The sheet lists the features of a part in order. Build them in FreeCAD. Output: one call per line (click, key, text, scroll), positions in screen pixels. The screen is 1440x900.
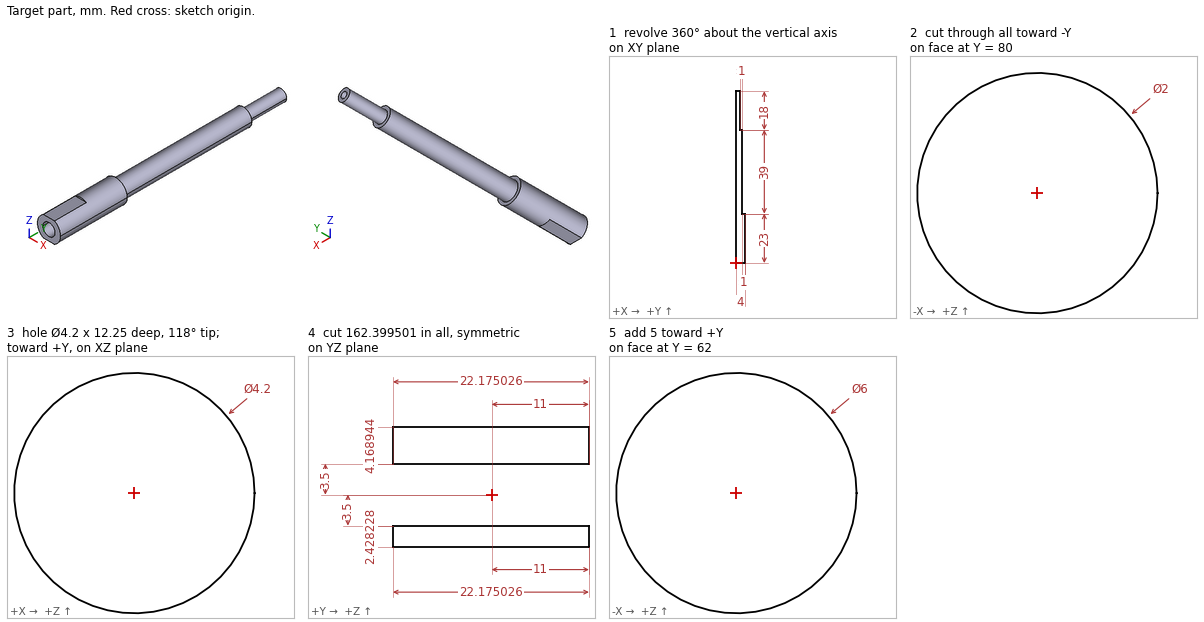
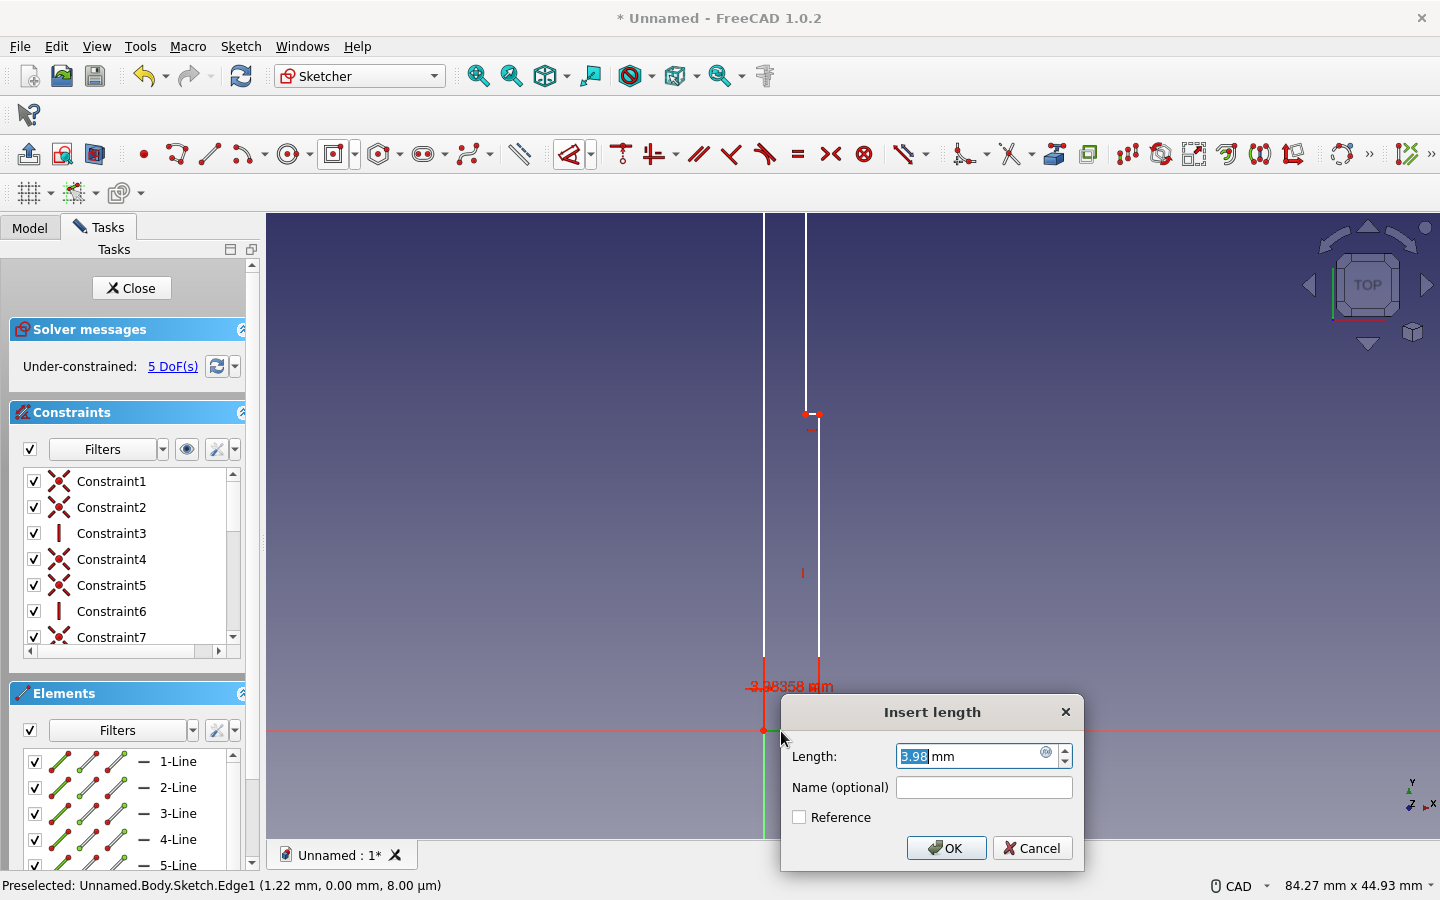
text(4)
key(Return)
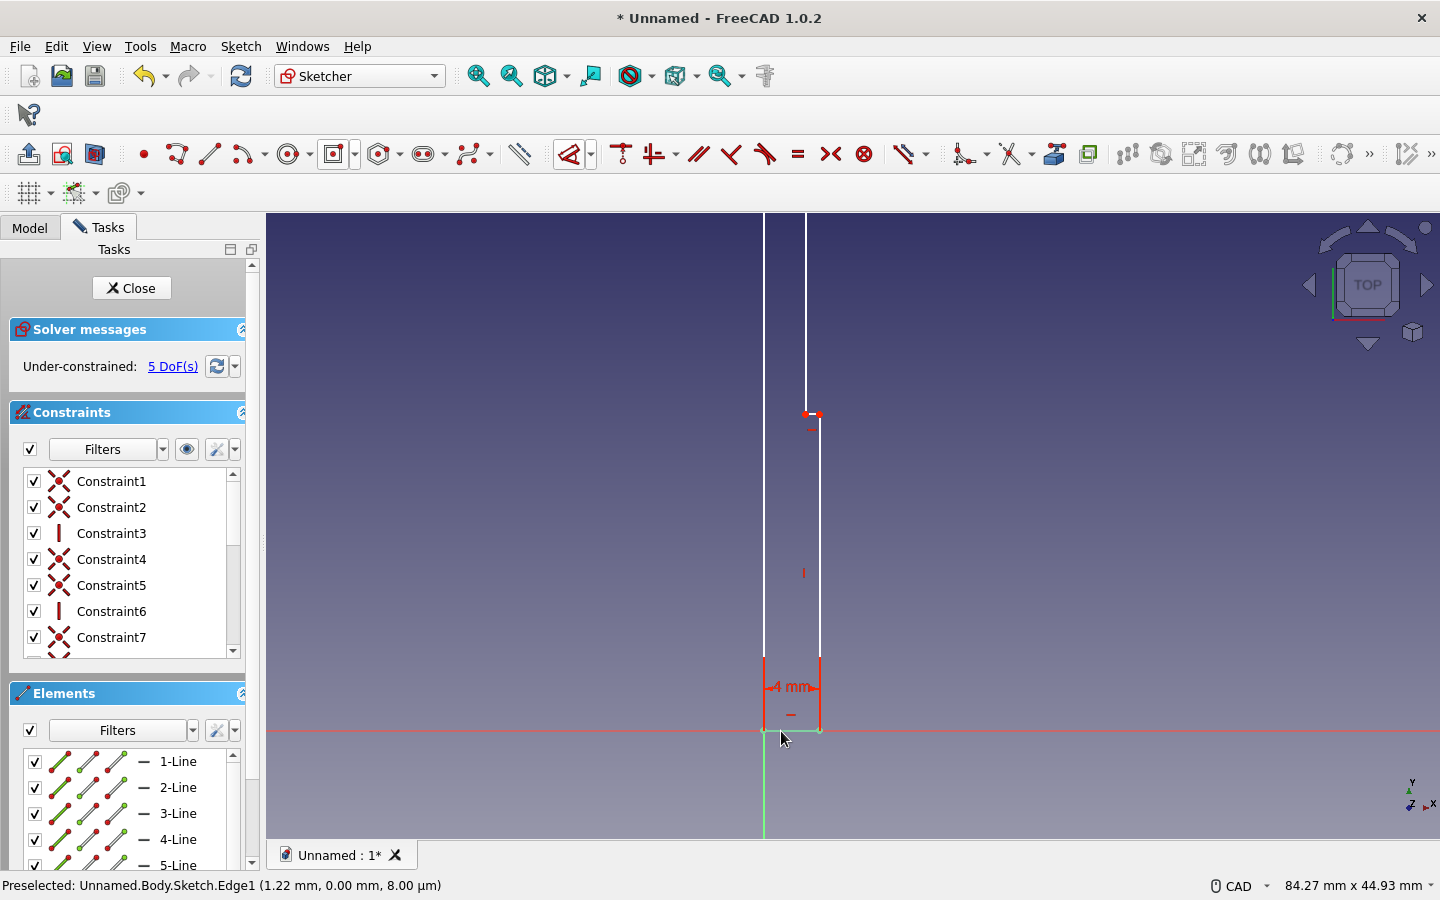
scroll(813, 414, up, 6)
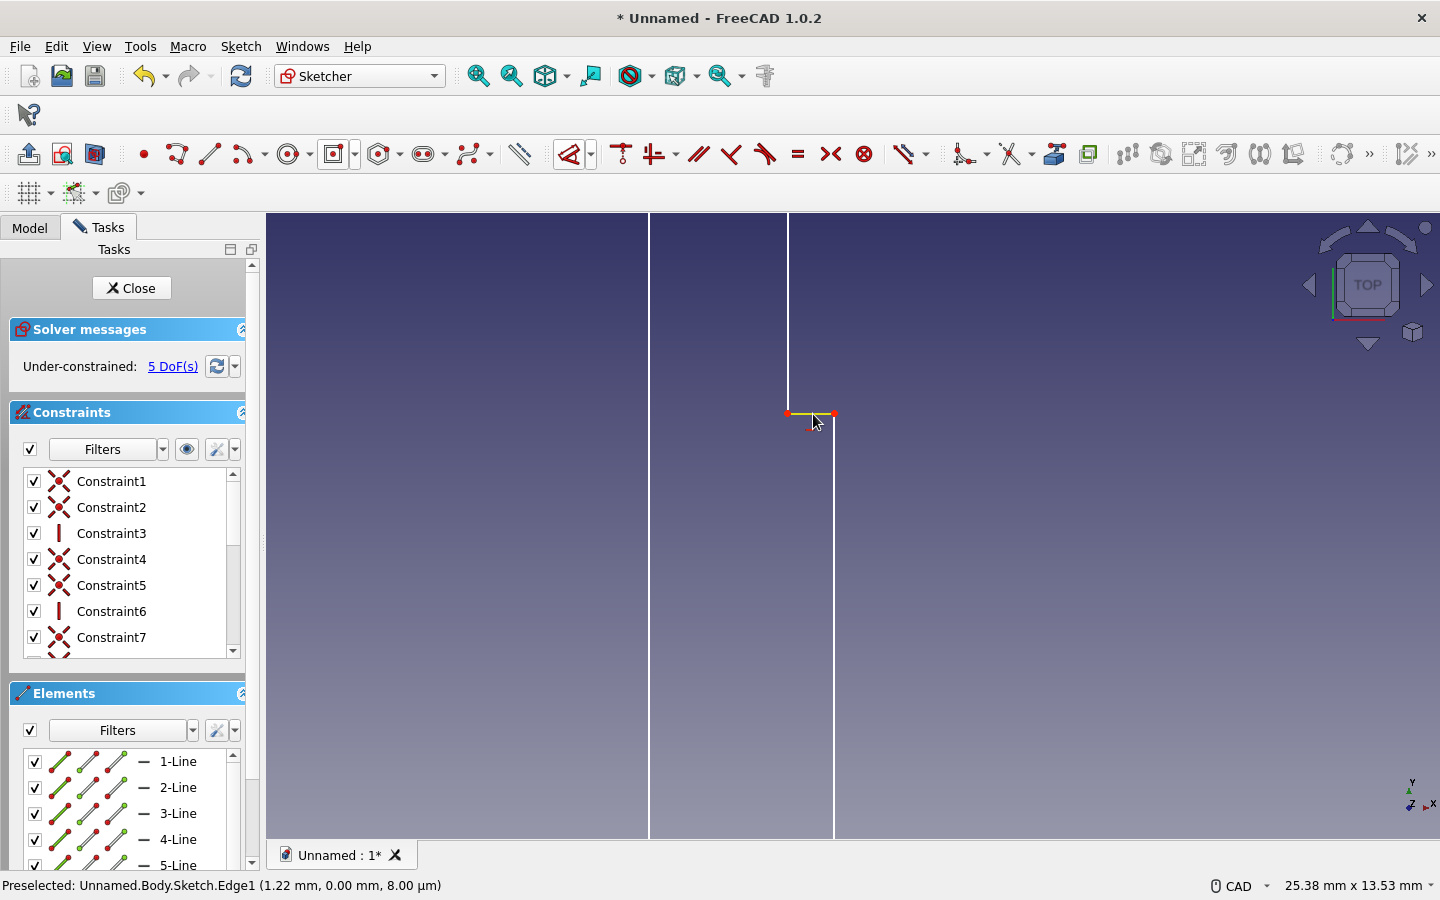
click(811, 414)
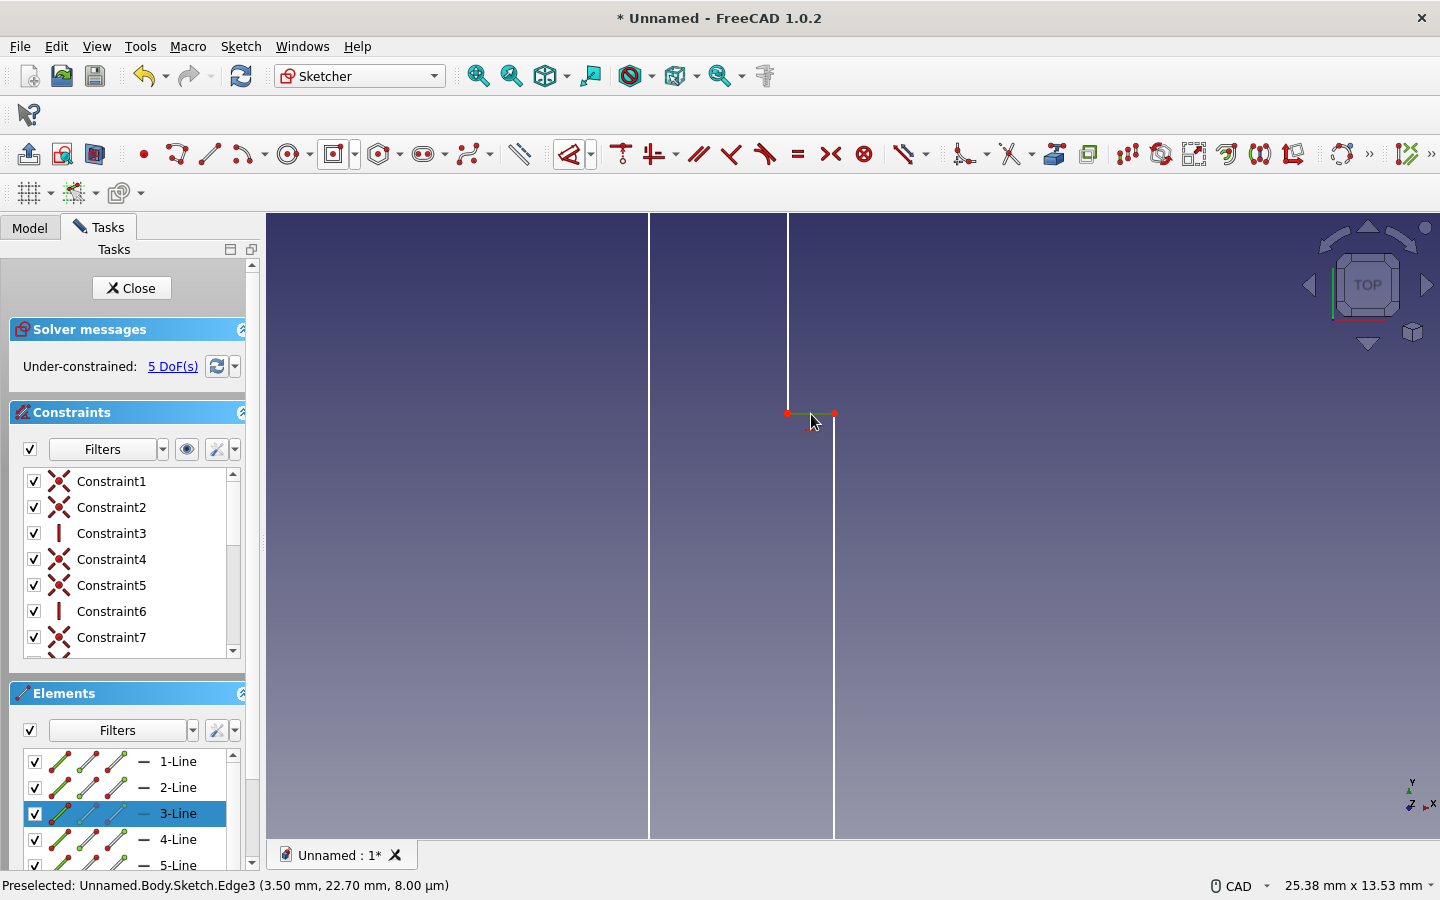
click(590, 154)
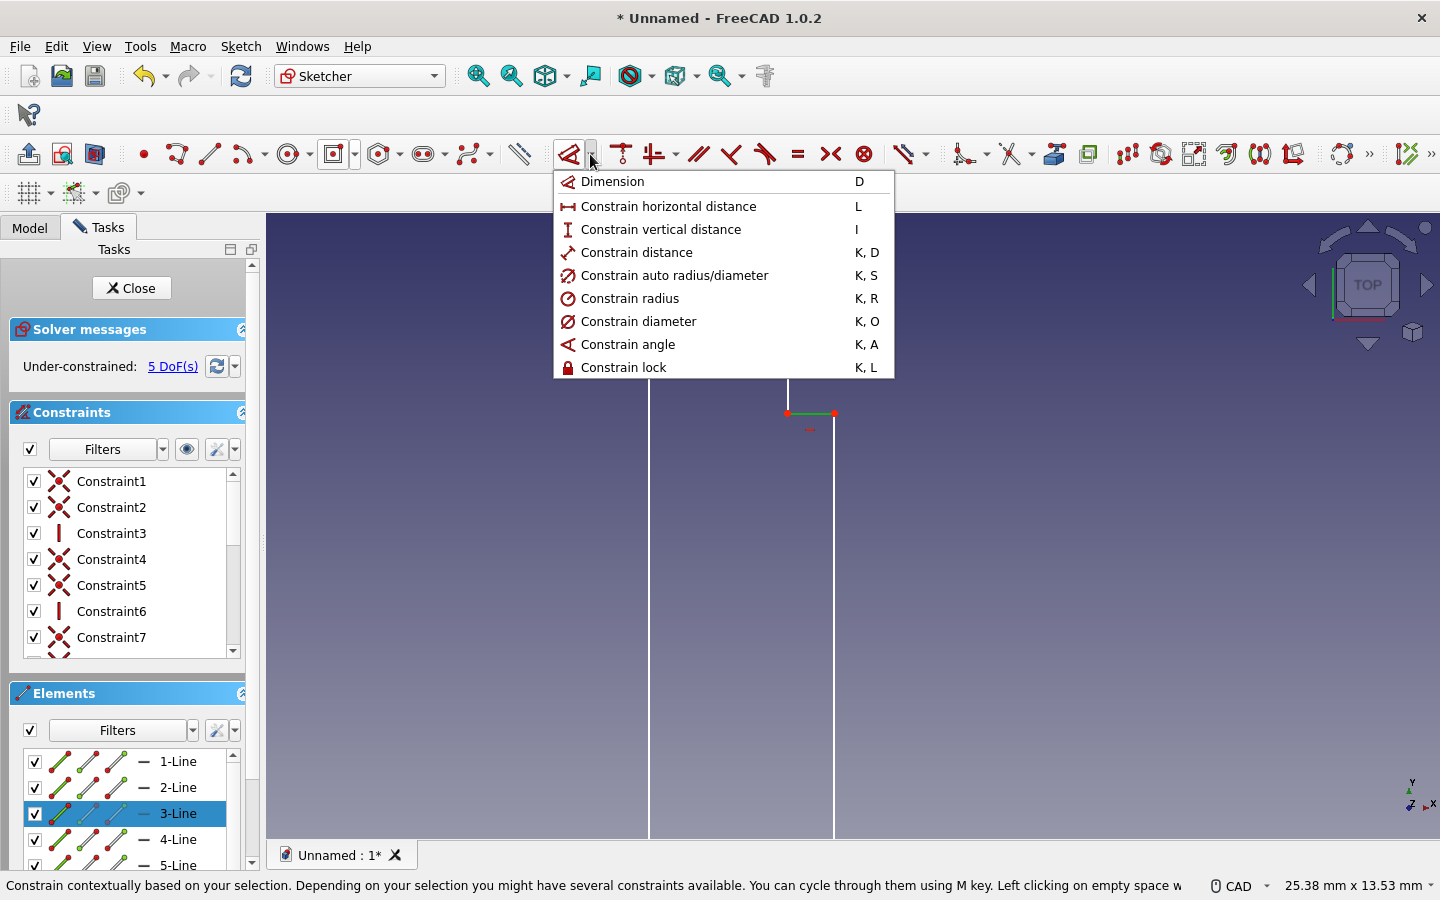
click(724, 206)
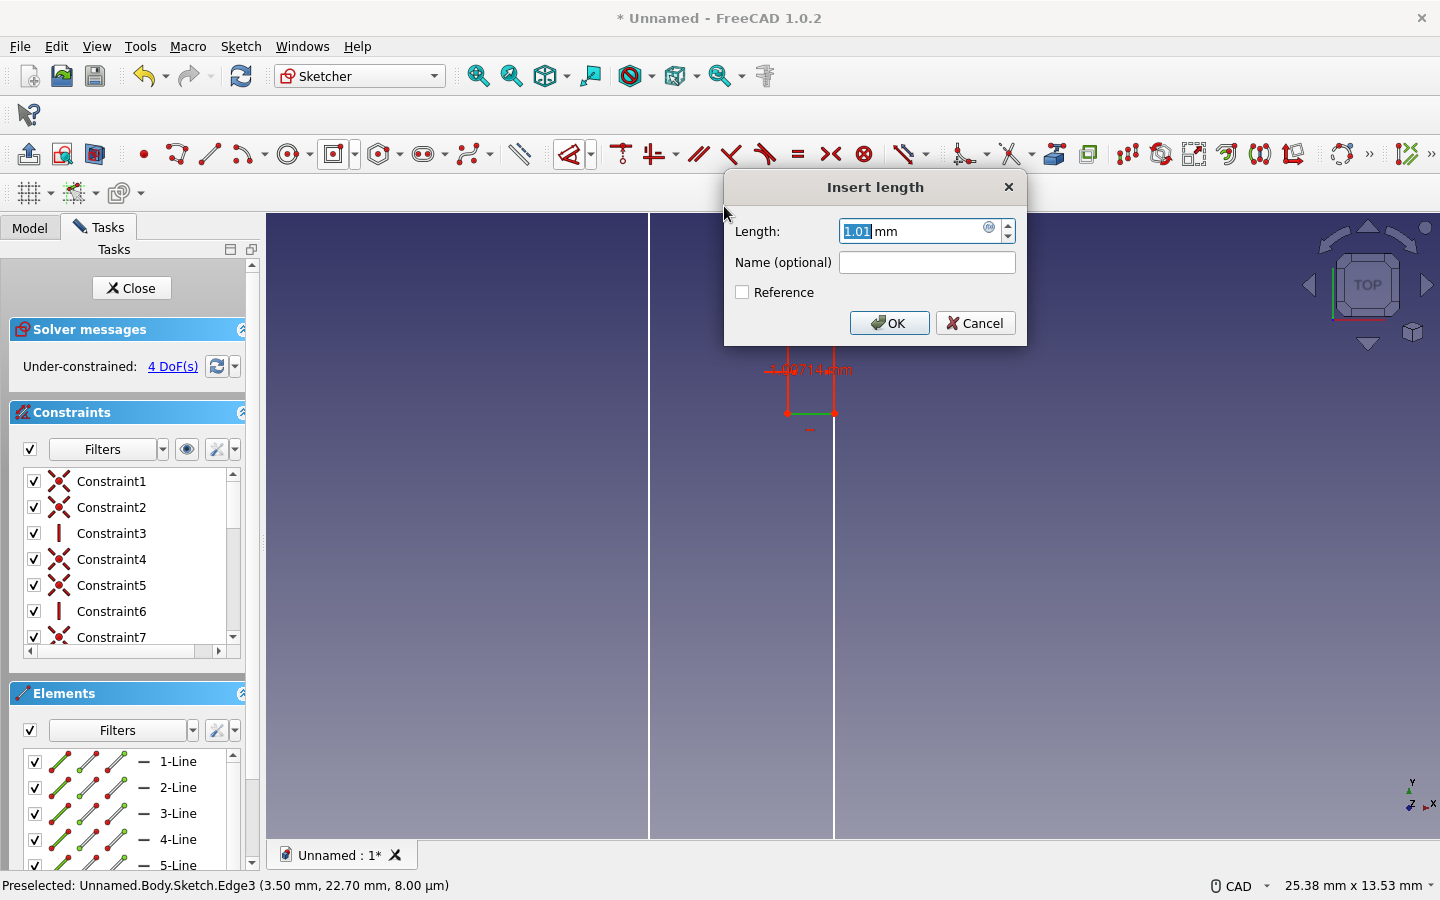
text(1)
key(Return)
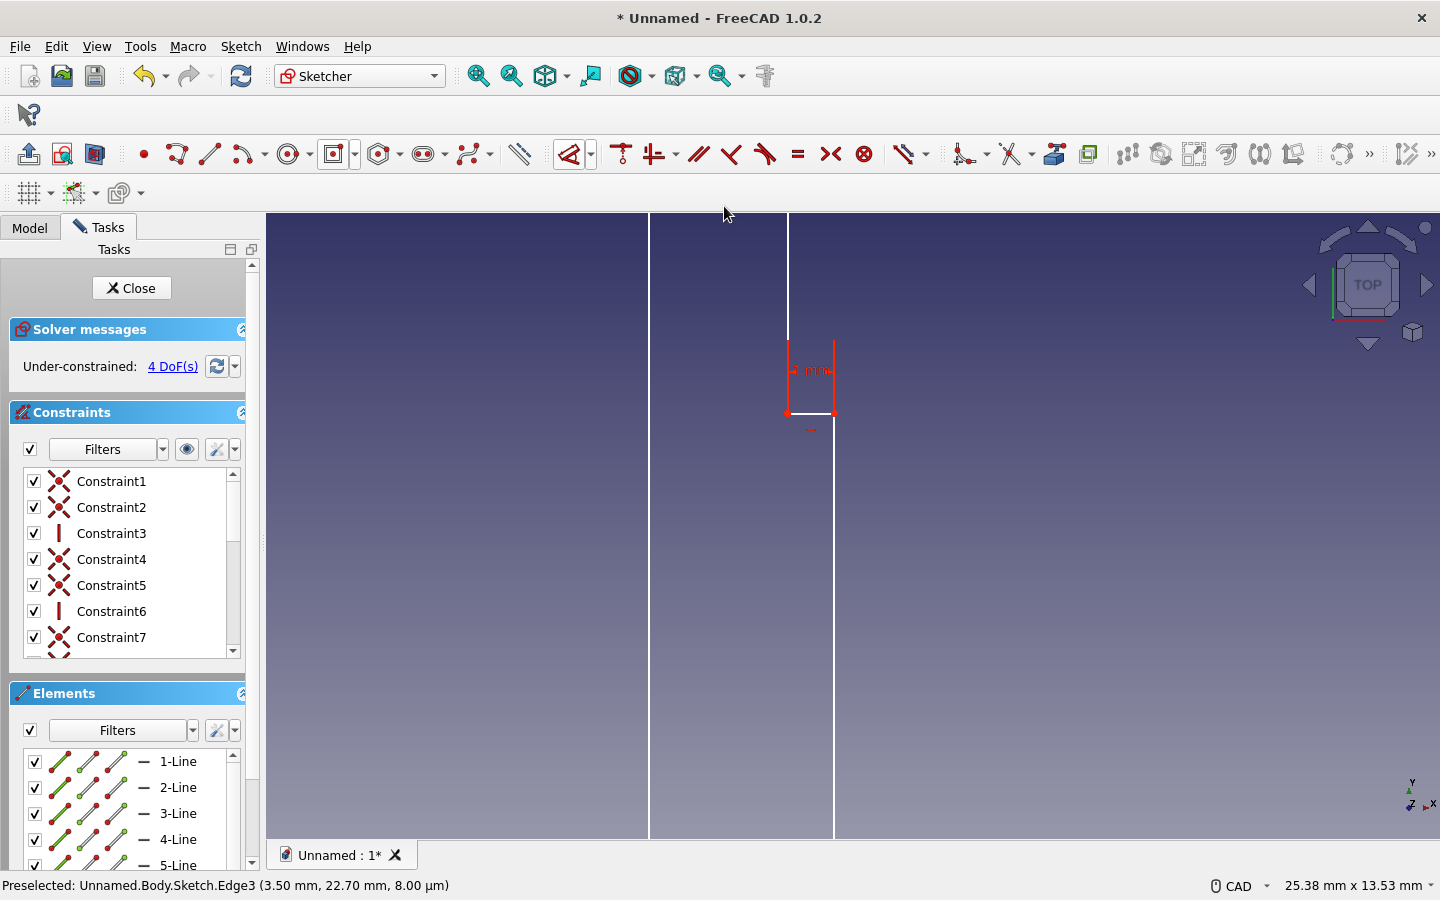
scroll(790, 640, down, 11)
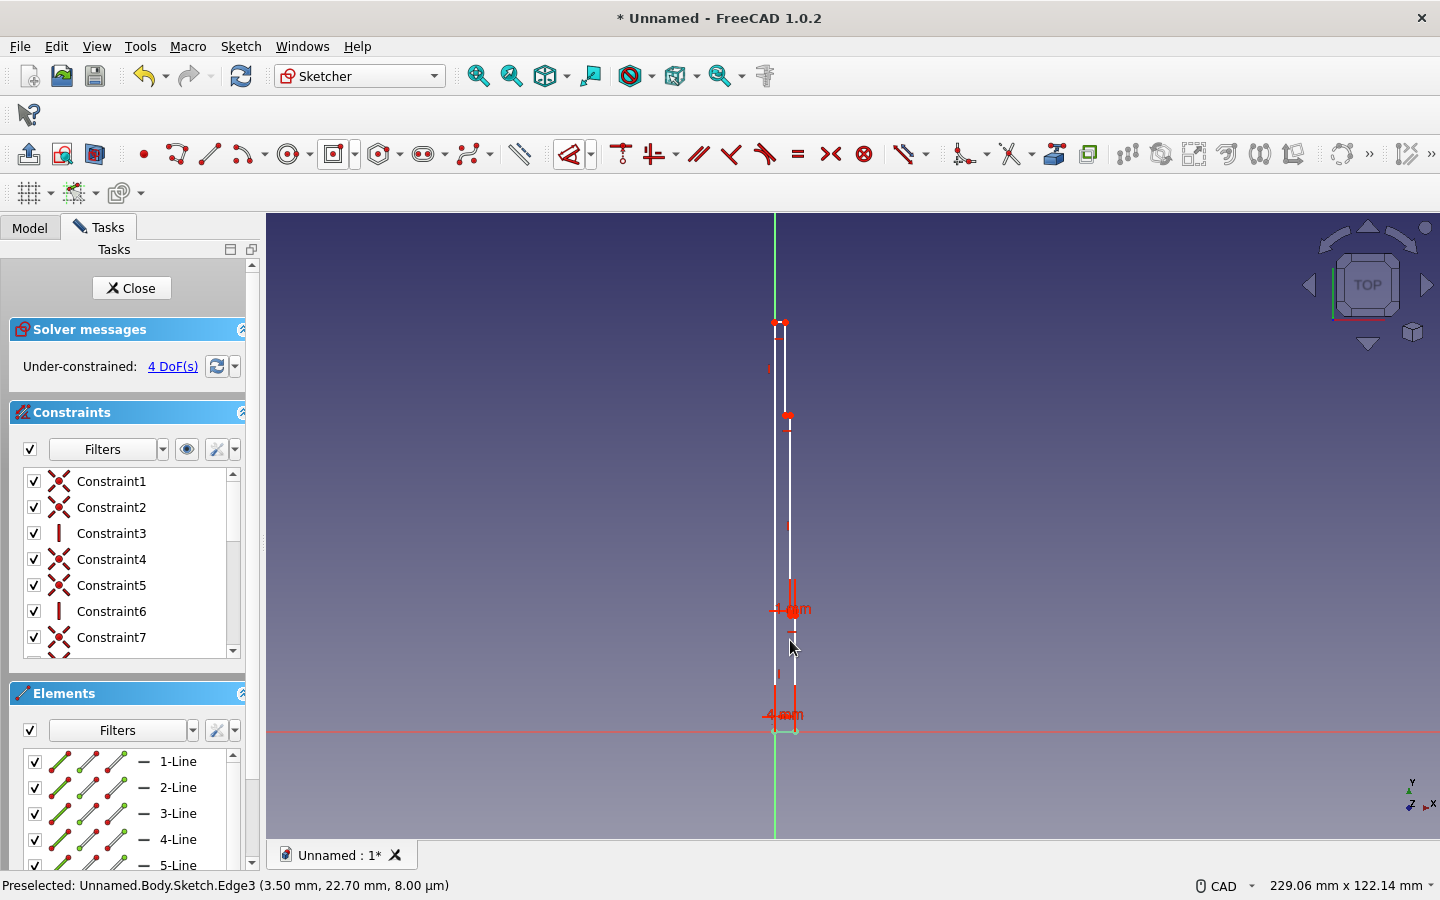
scroll(789, 415, up, 11)